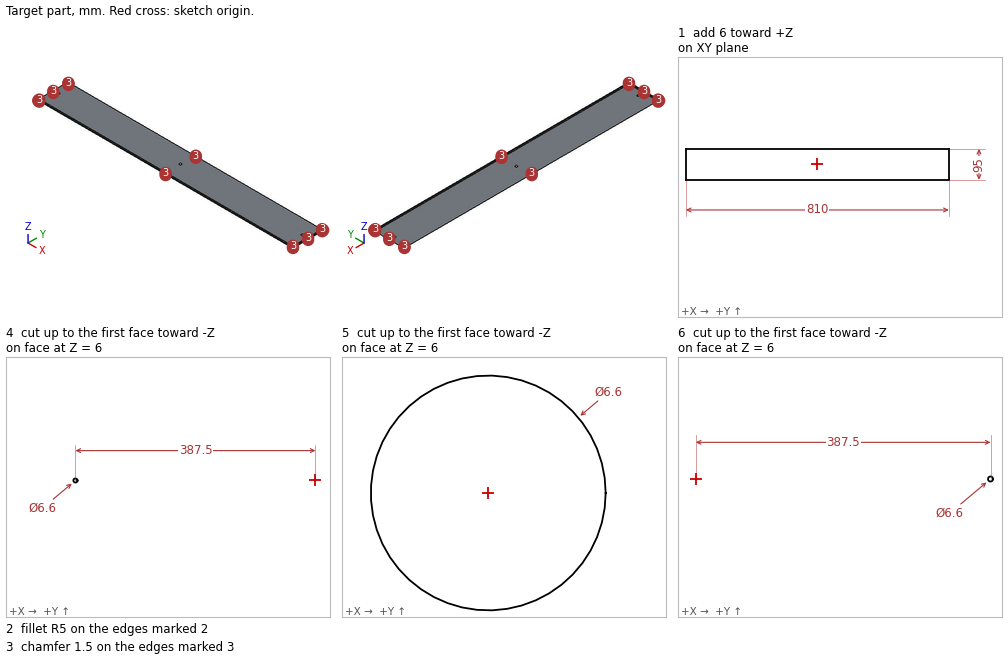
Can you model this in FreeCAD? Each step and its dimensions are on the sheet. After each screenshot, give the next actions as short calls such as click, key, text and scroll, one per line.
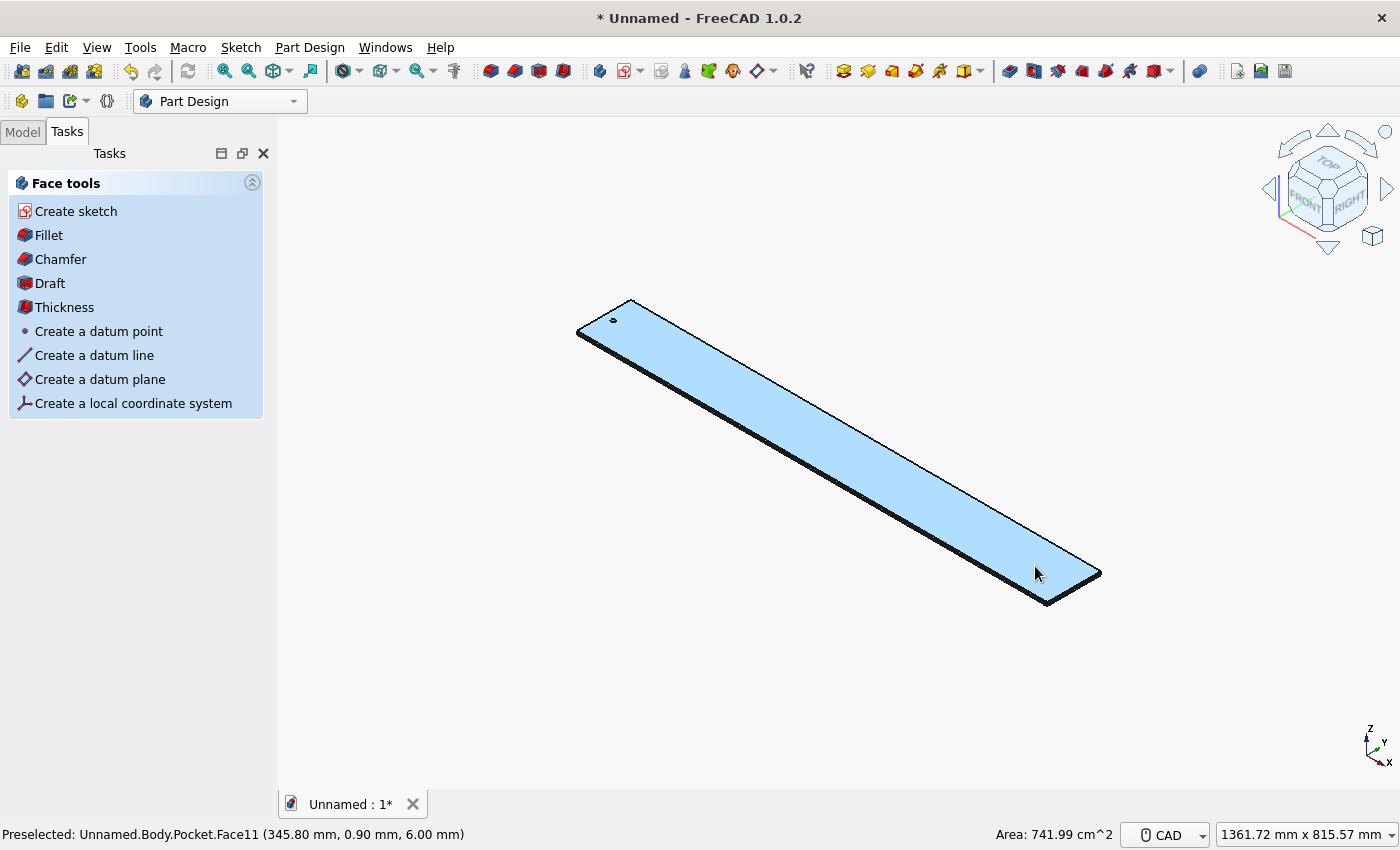
click(624, 72)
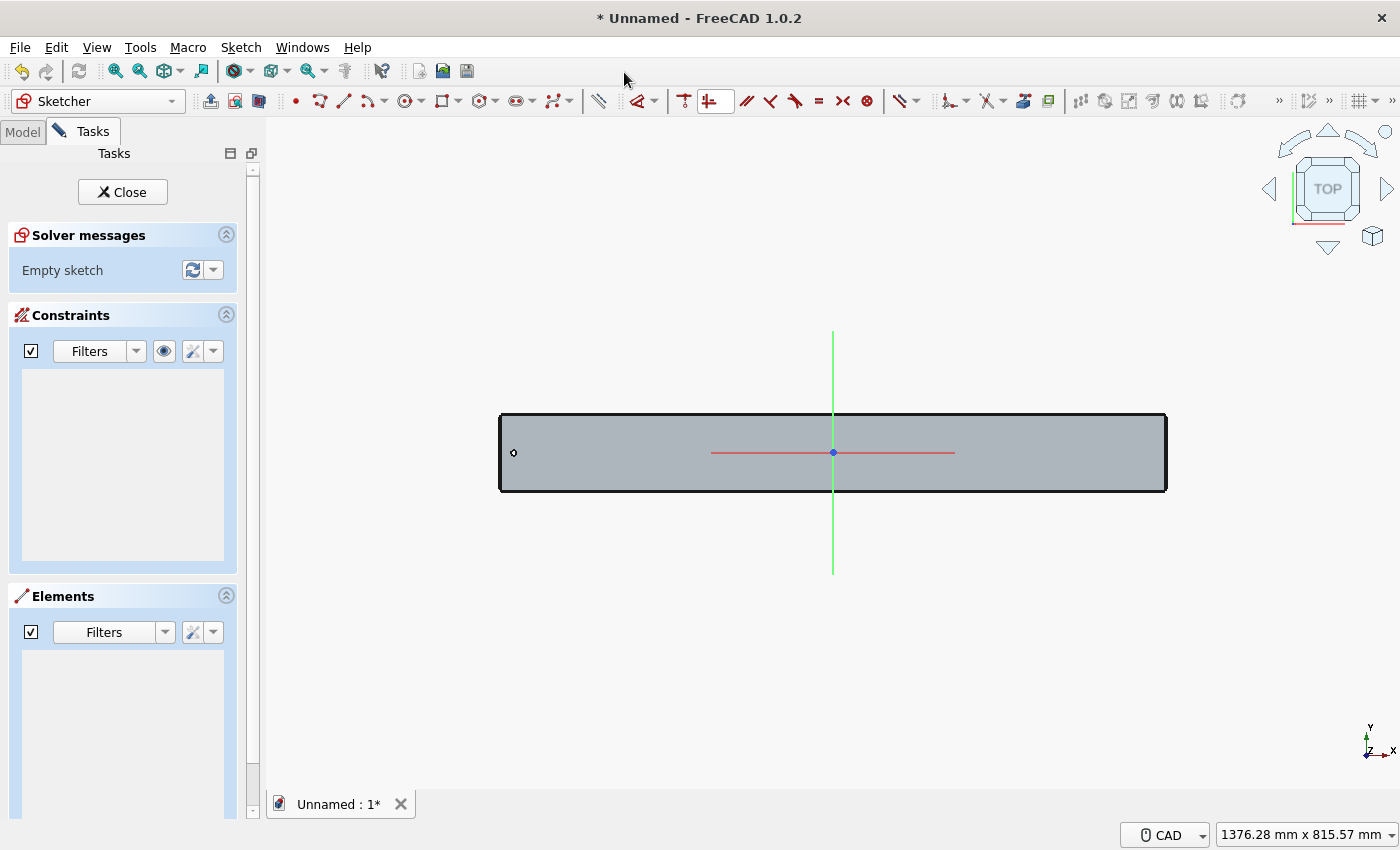
scroll(837, 453, up, 15)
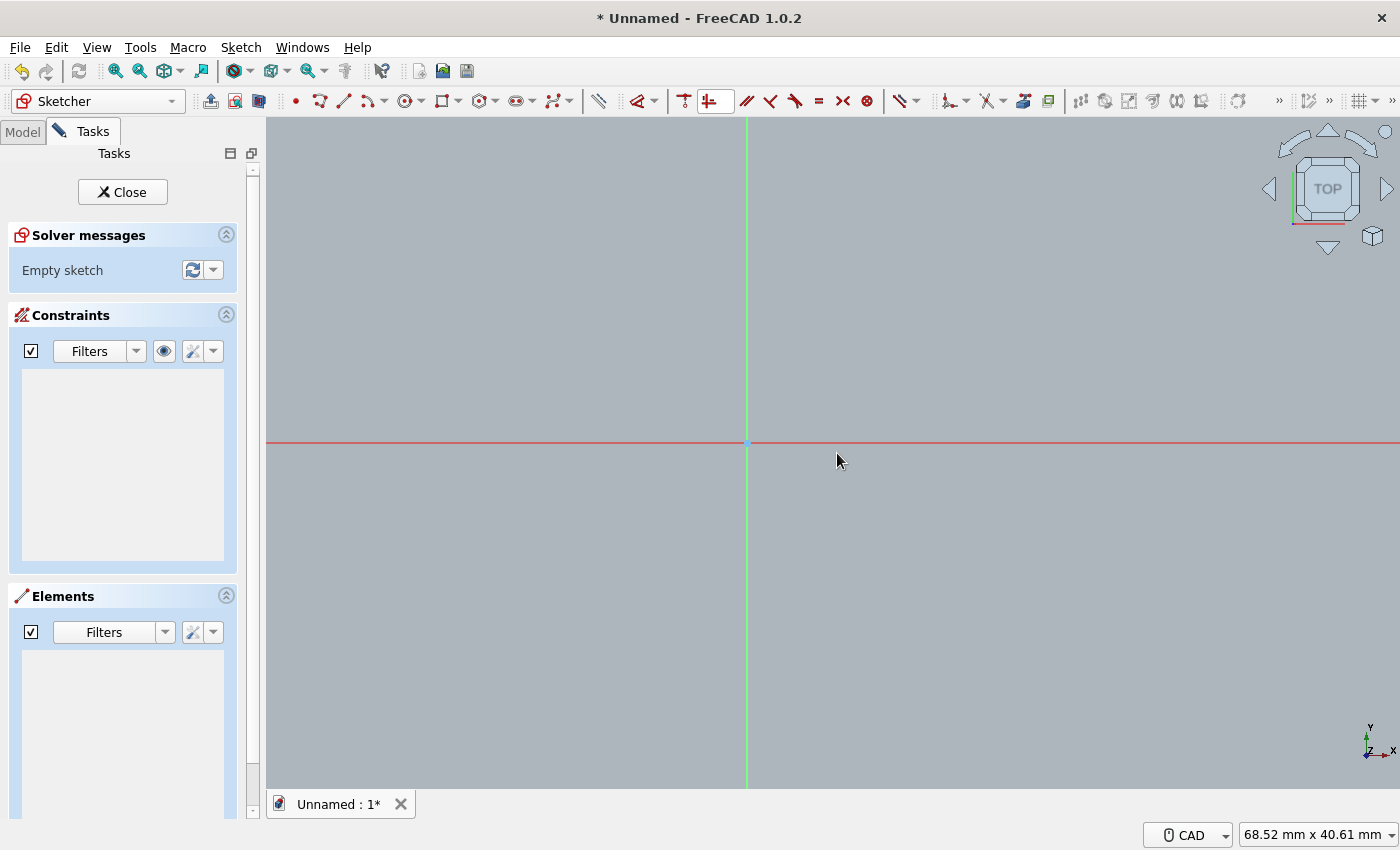
scroll(741, 440, up, 7)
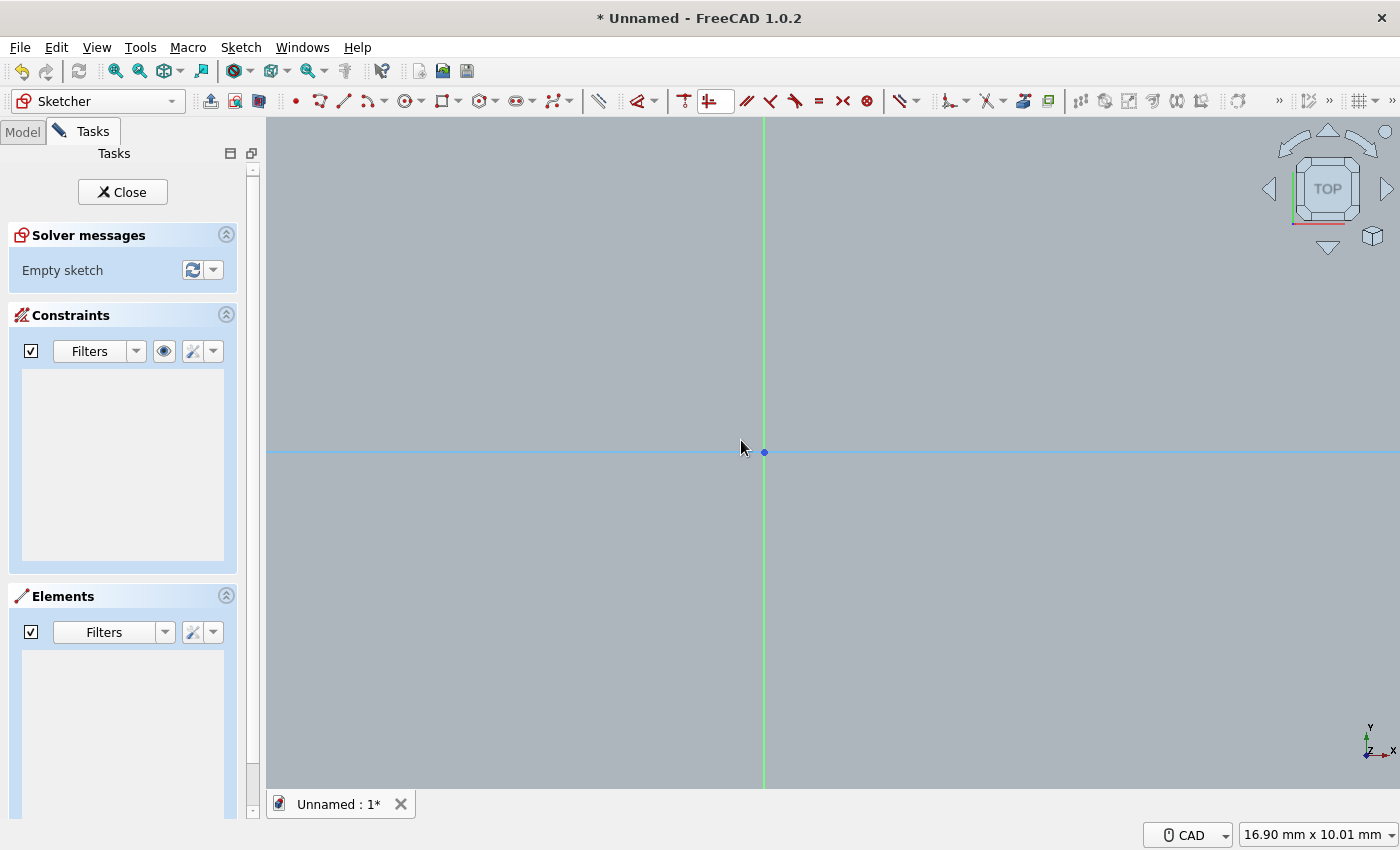
key(g)
key(c)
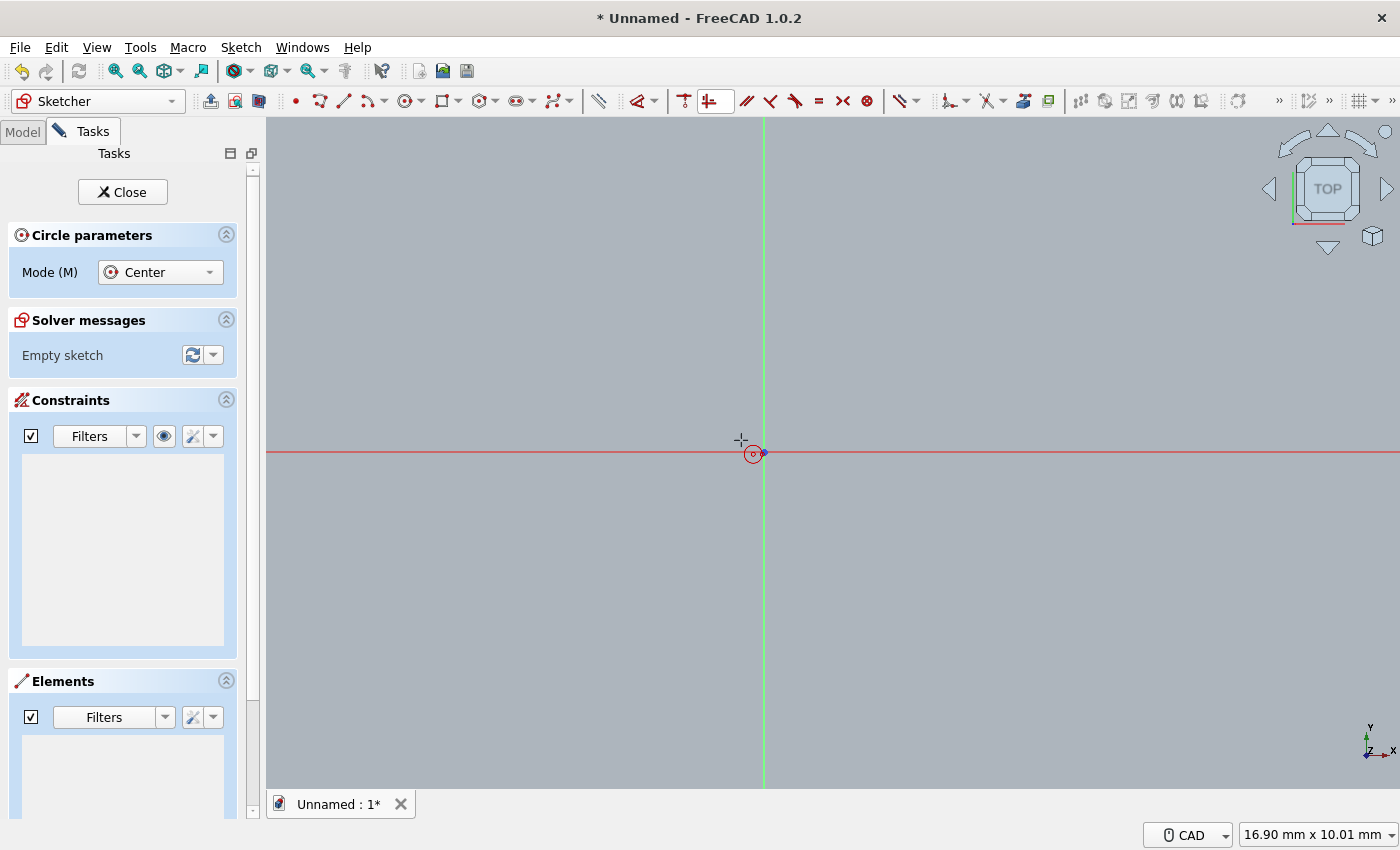
click(764, 452)
move(921, 296)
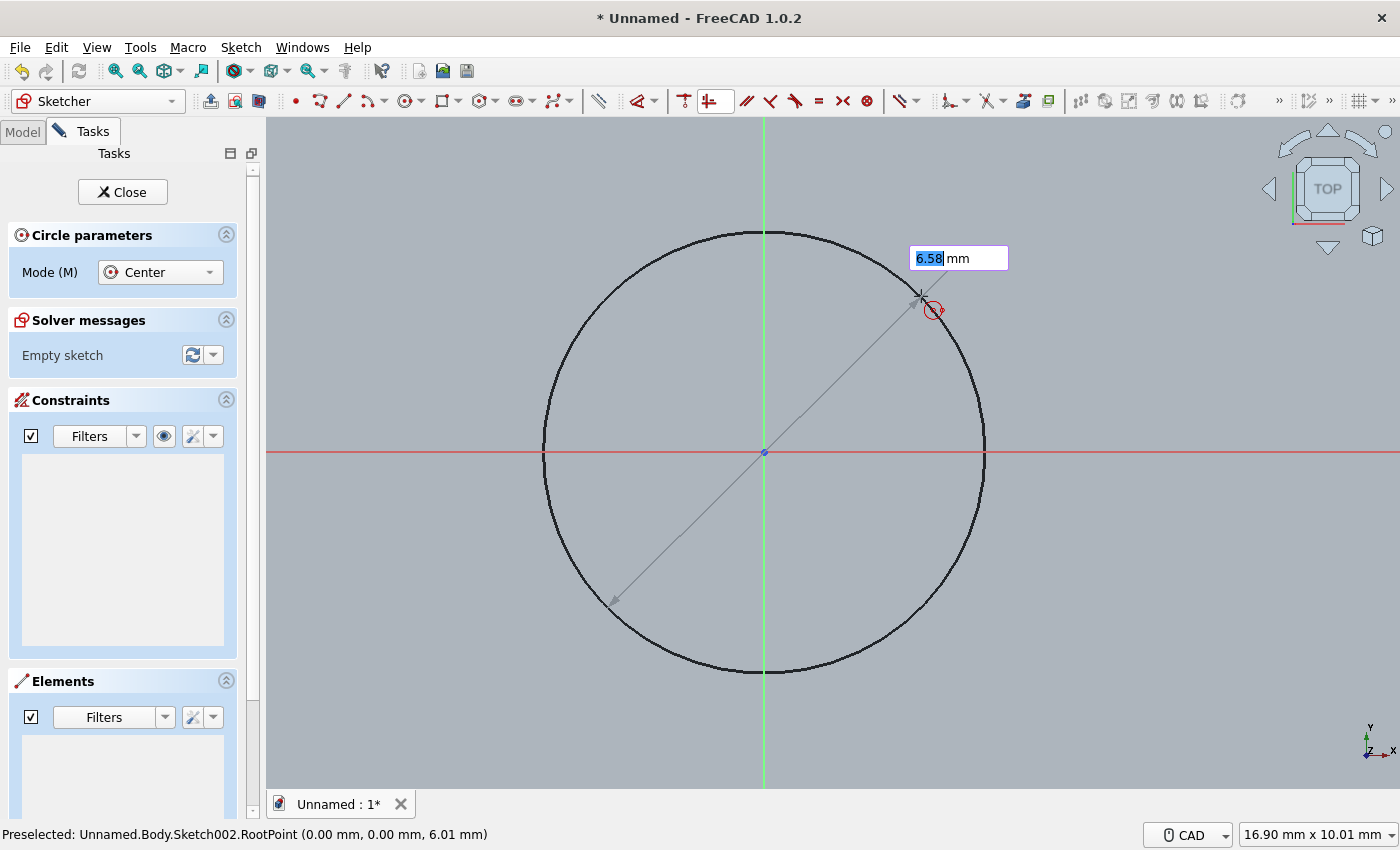
text(6.6)
key(Return)
key(Escape)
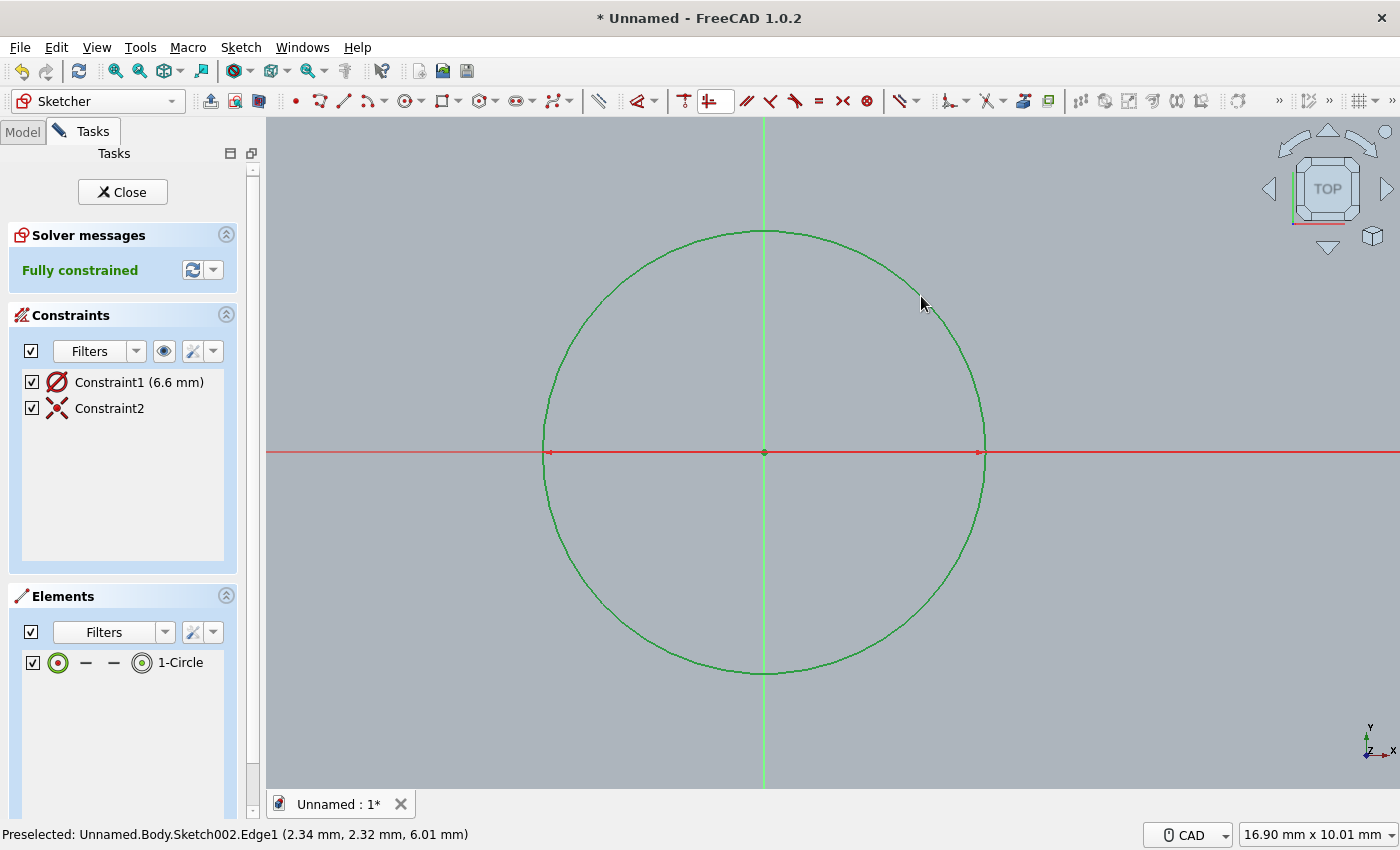
click(123, 192)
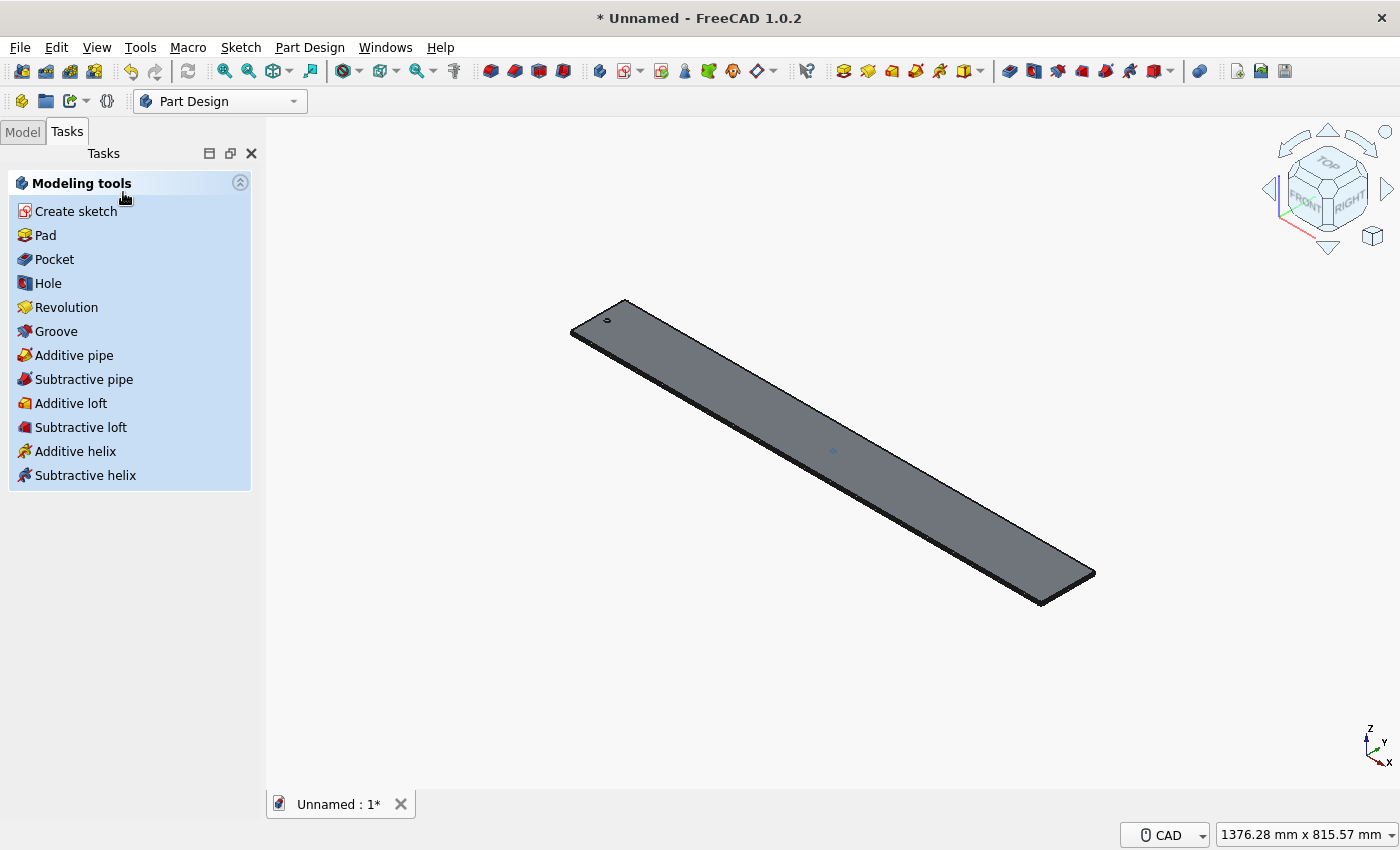
click(1010, 72)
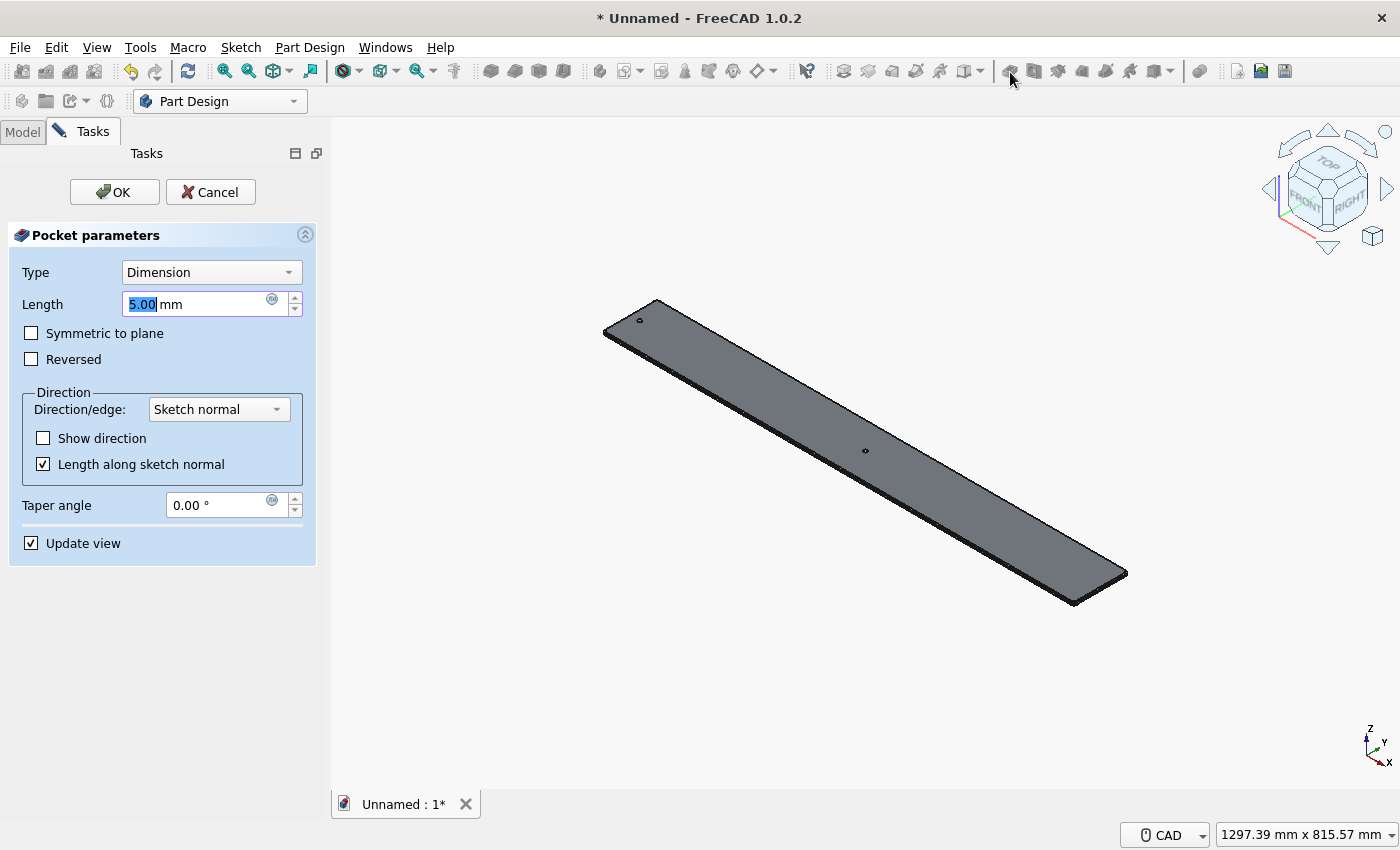
click(212, 272)